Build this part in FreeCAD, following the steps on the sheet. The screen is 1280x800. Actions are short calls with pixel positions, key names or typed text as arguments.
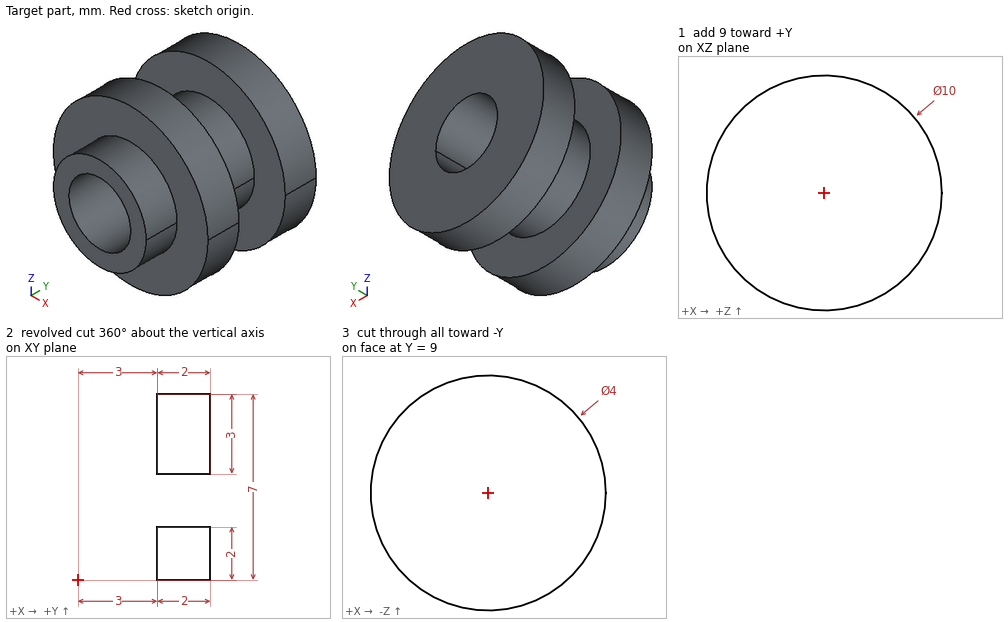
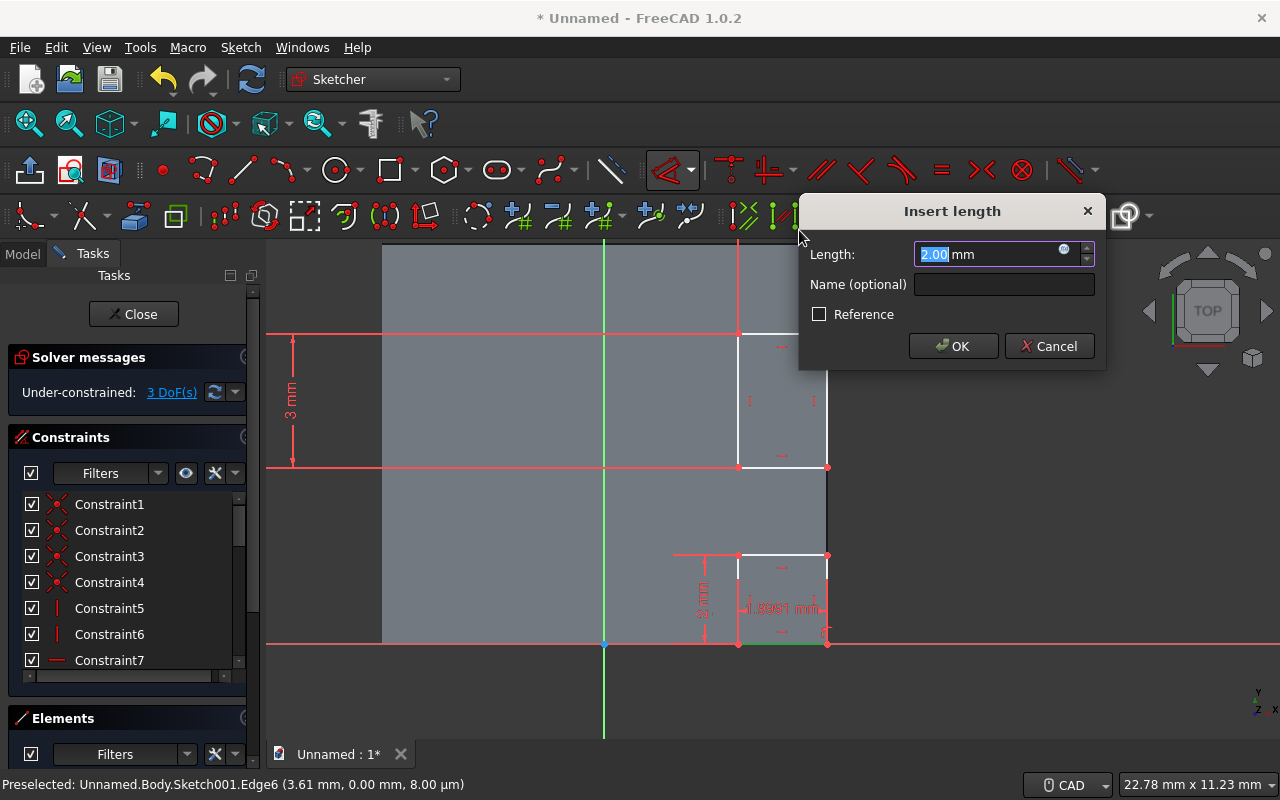
text(2)
key(Return)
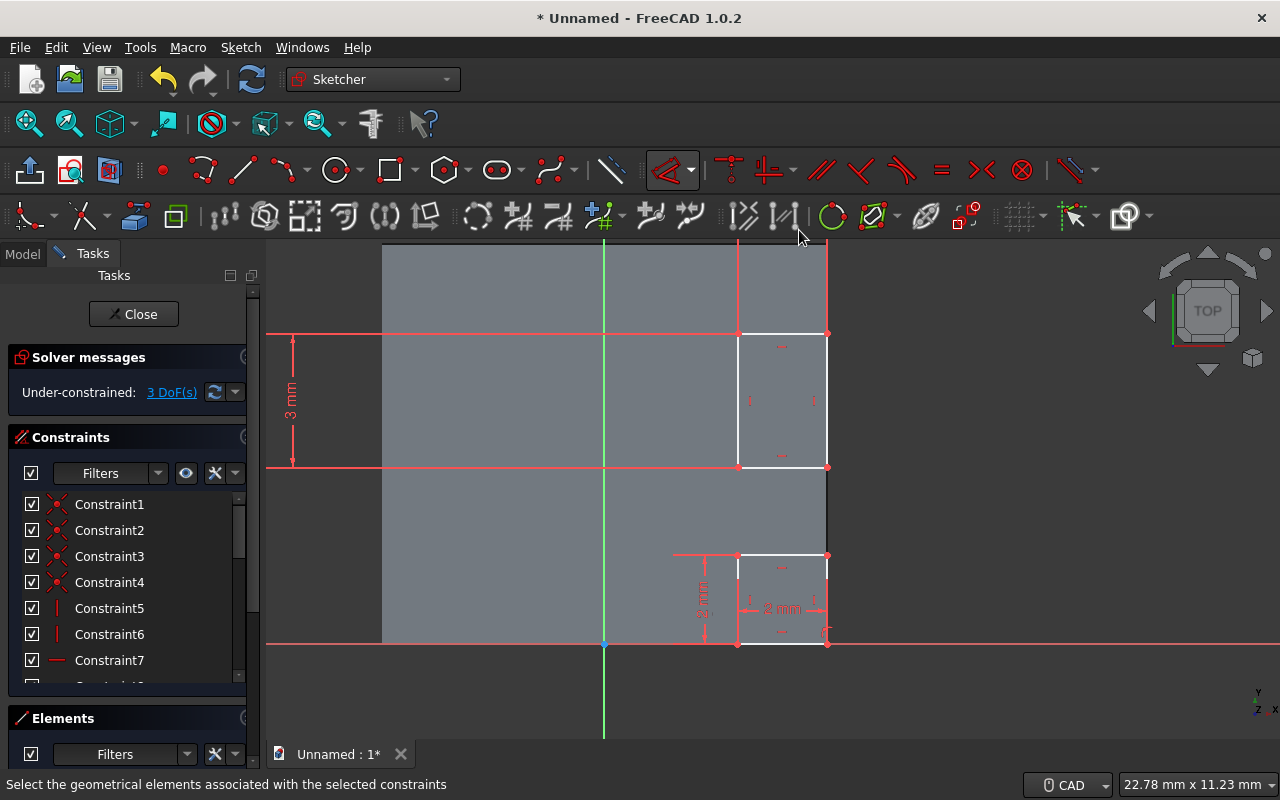
click(738, 334)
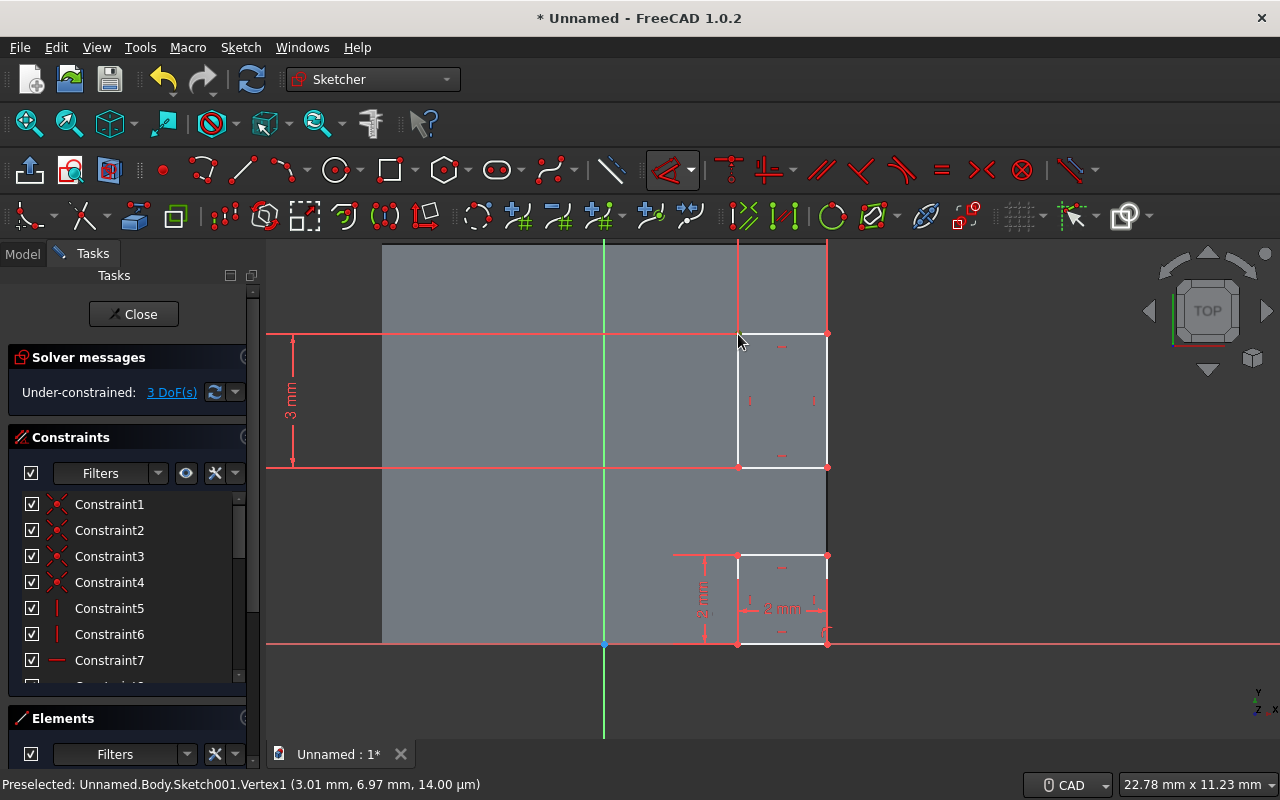
key(l)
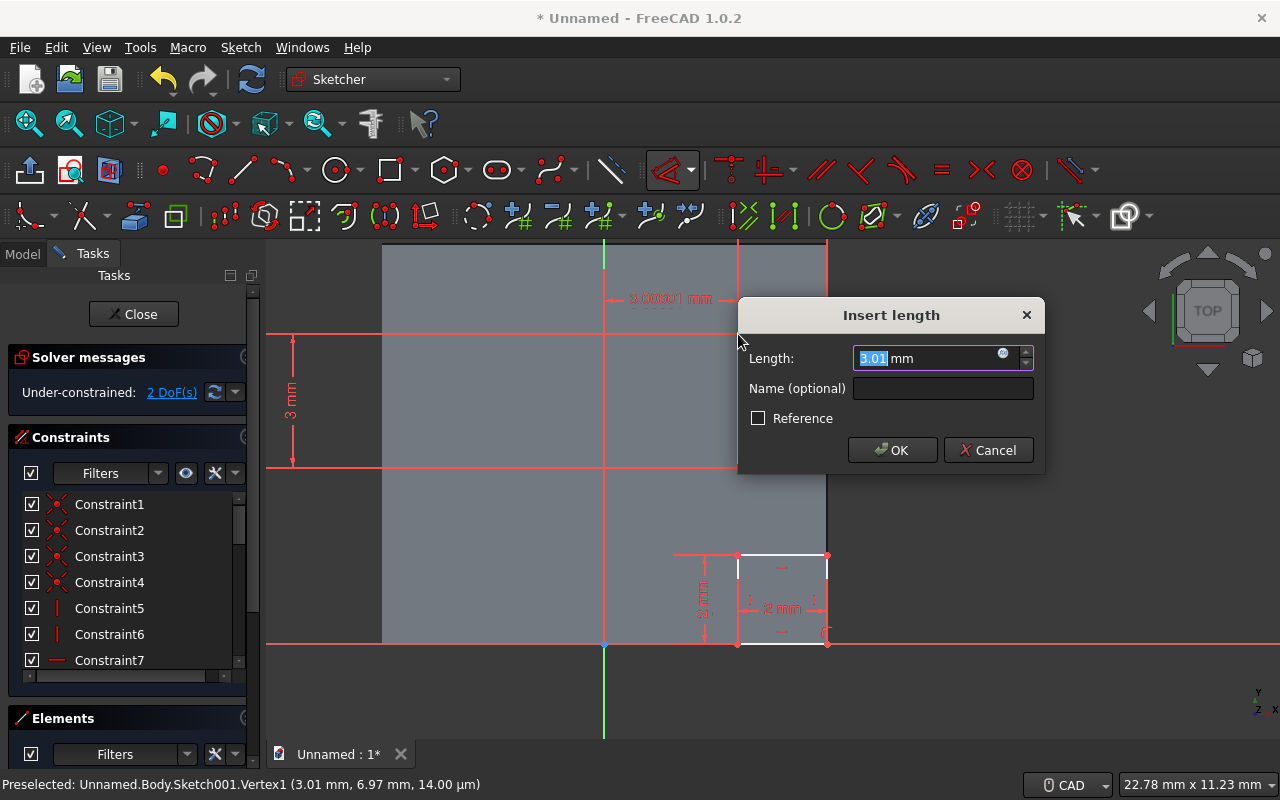
text(3)
key(Return)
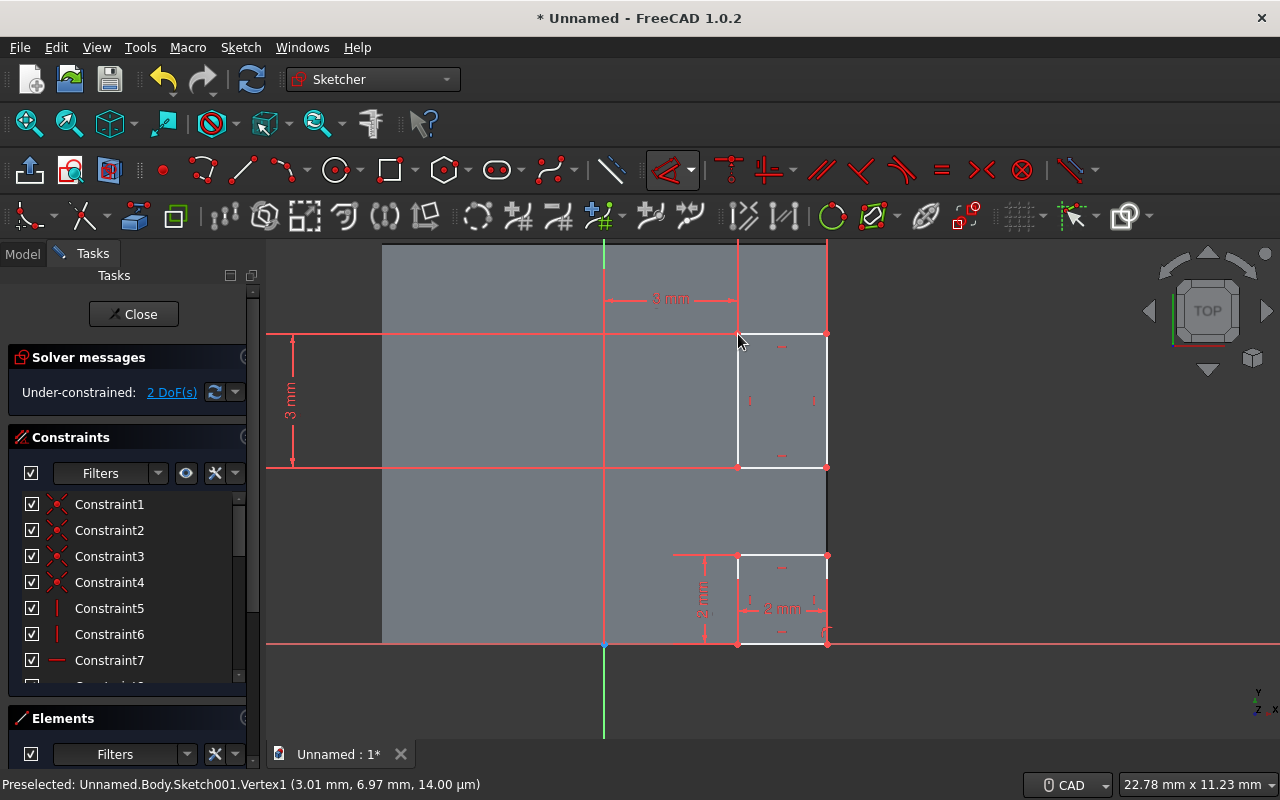
click(738, 334)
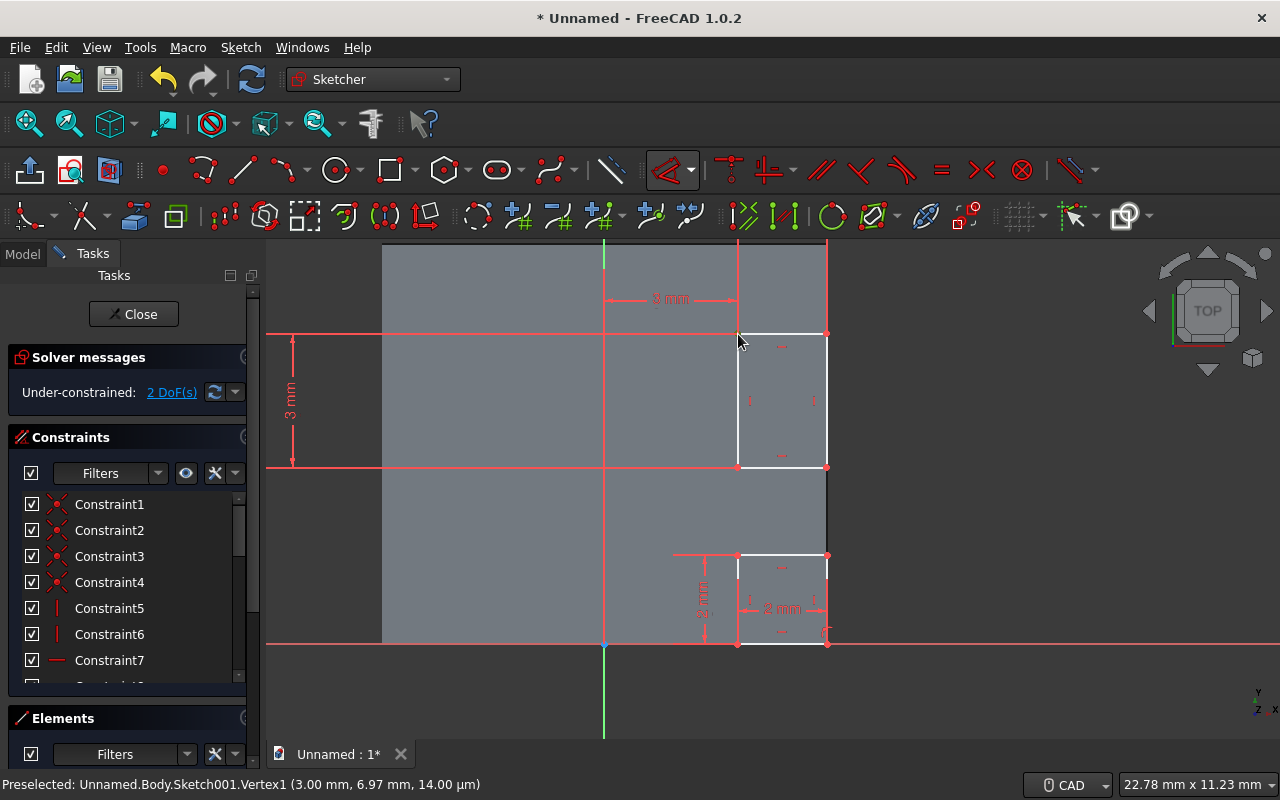
click(694, 170)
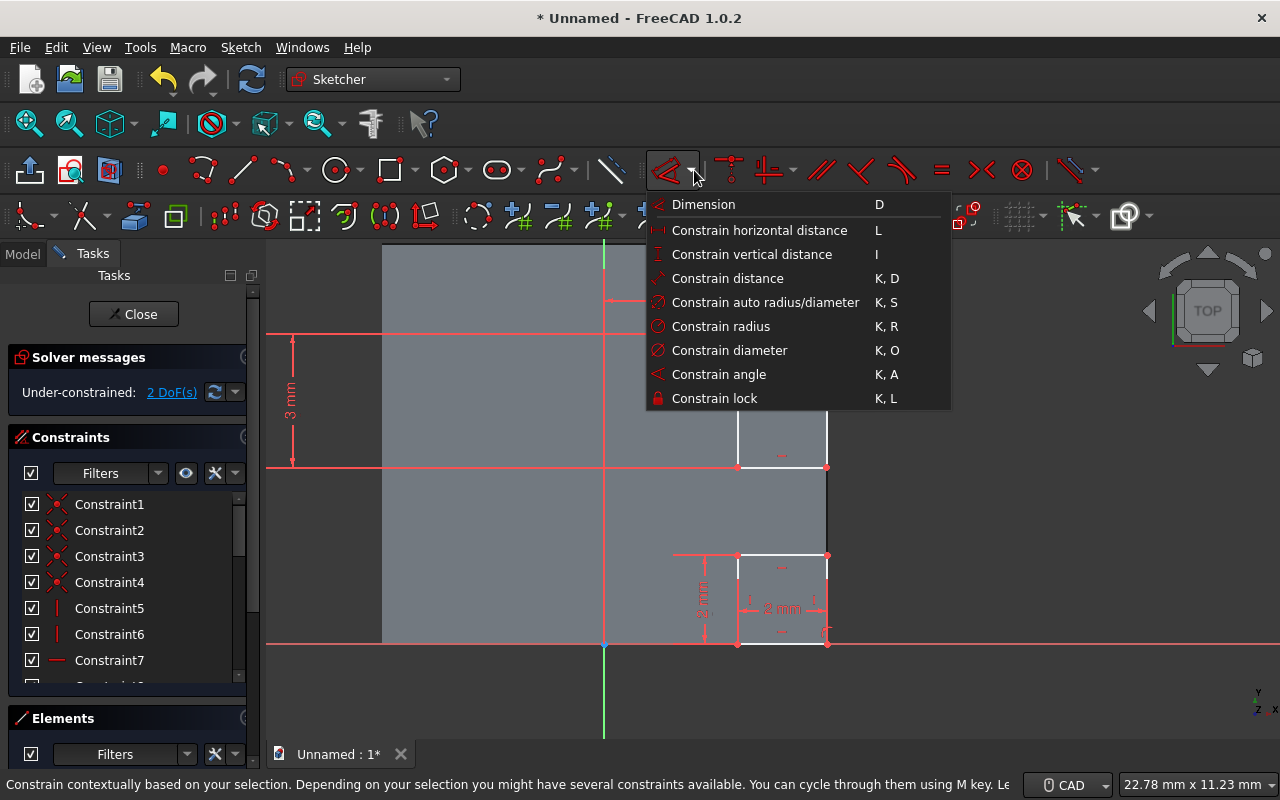
click(799, 254)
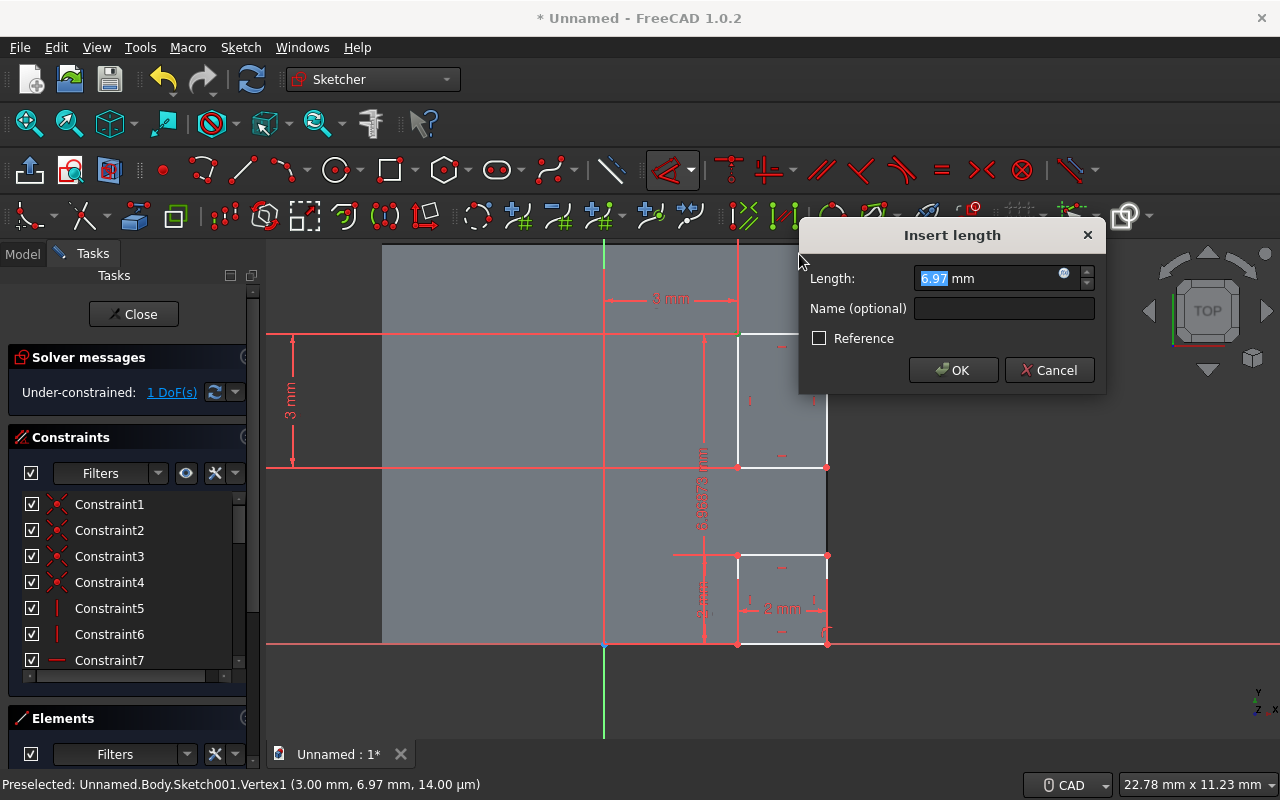
text(7)
key(Return)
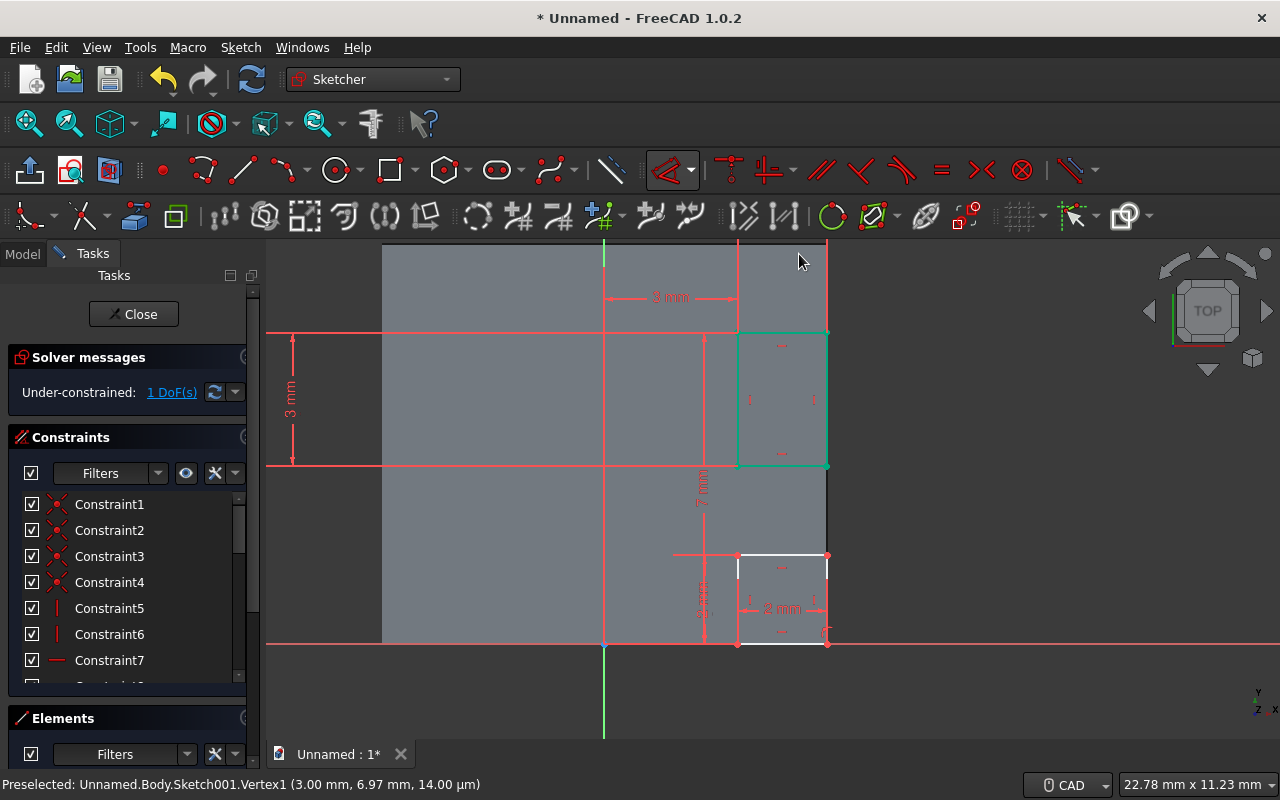
click(738, 555)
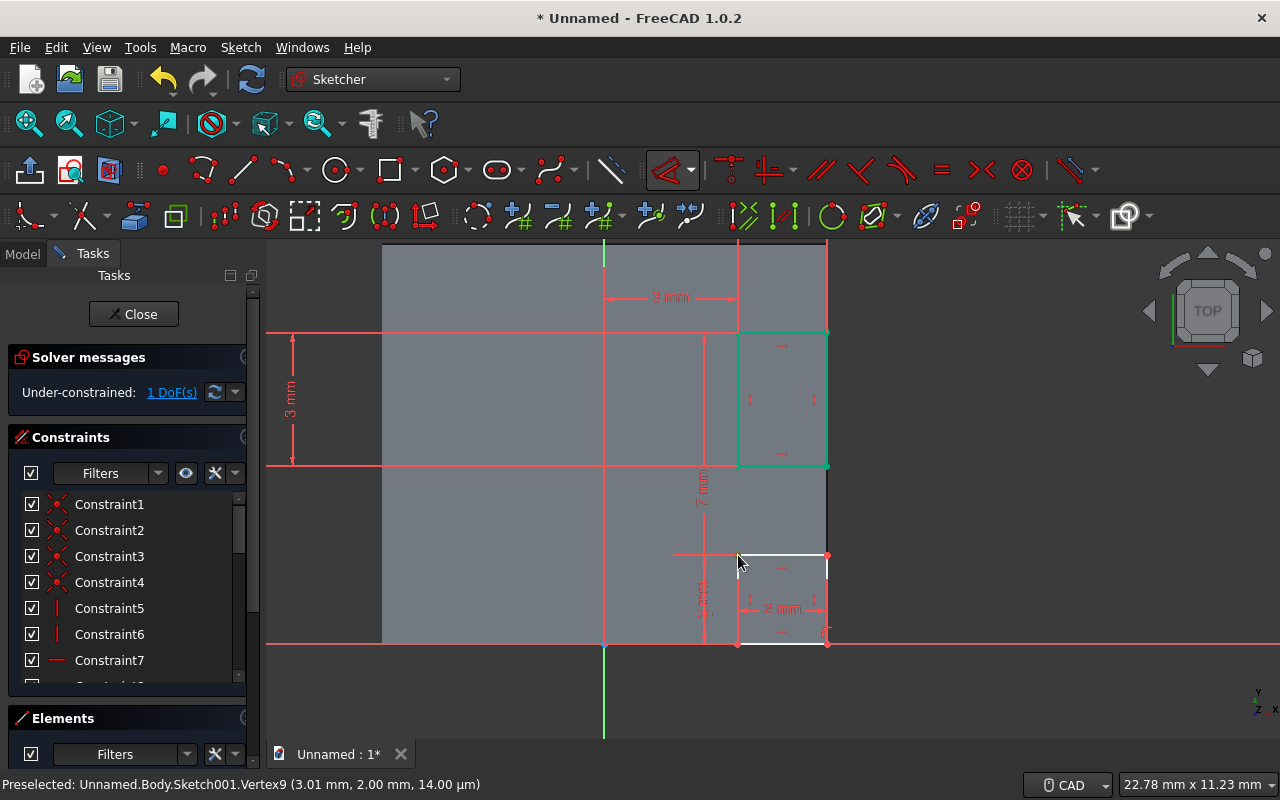
key(l)